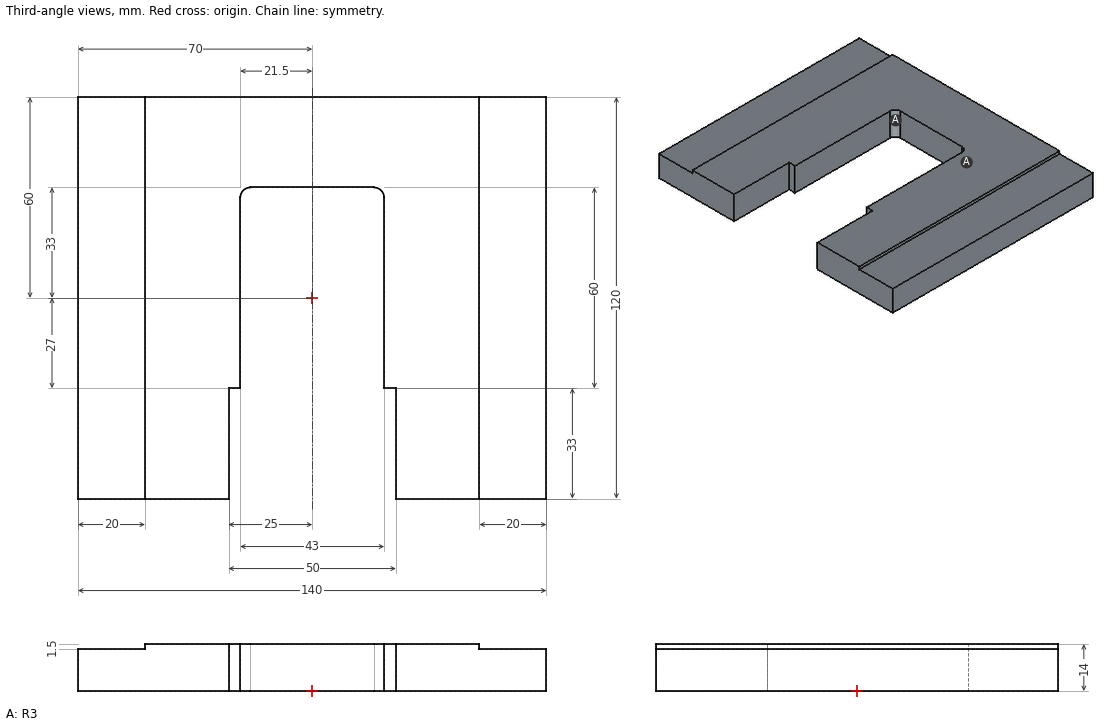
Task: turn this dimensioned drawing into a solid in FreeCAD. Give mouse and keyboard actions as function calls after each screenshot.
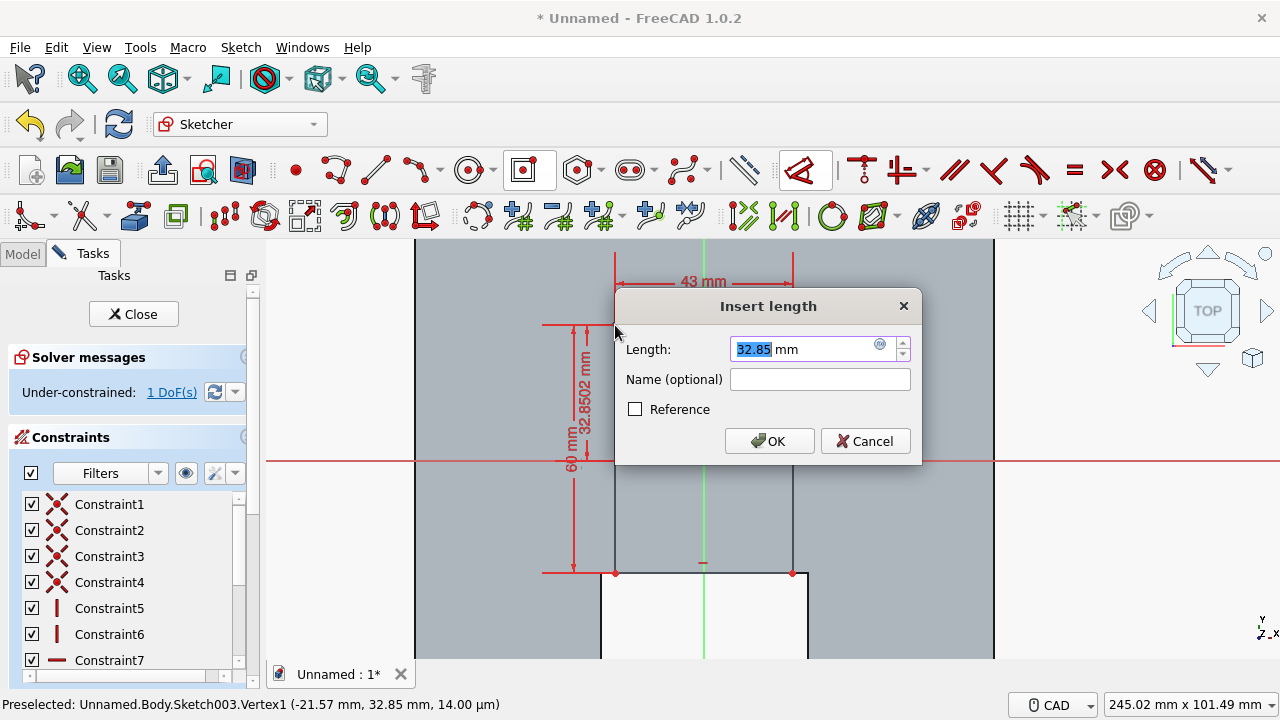
text(33)
key(Return)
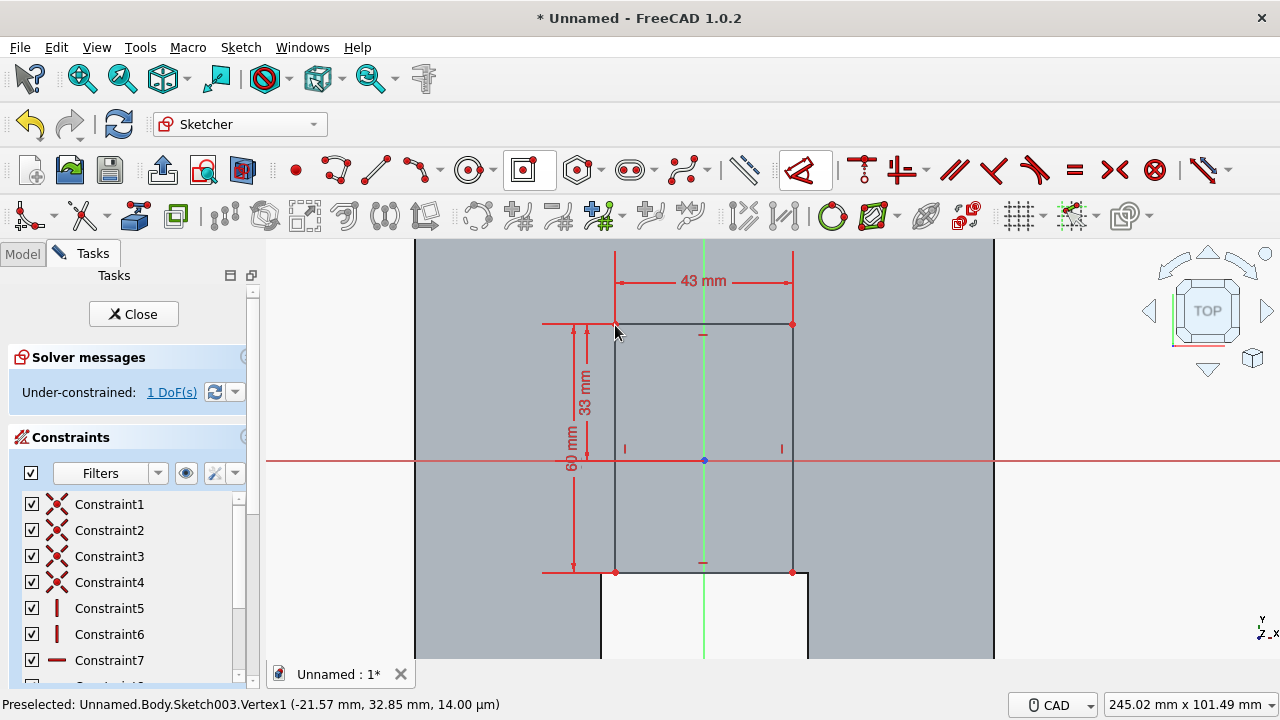
click(615, 324)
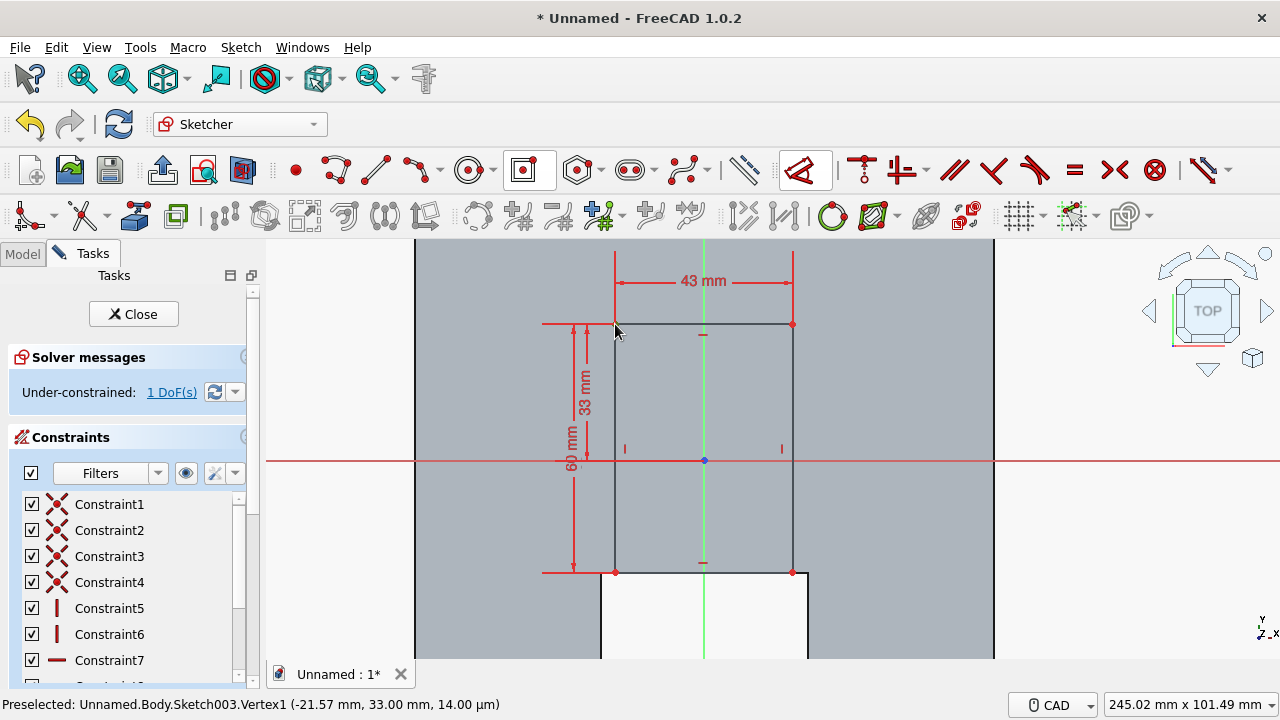
key(l)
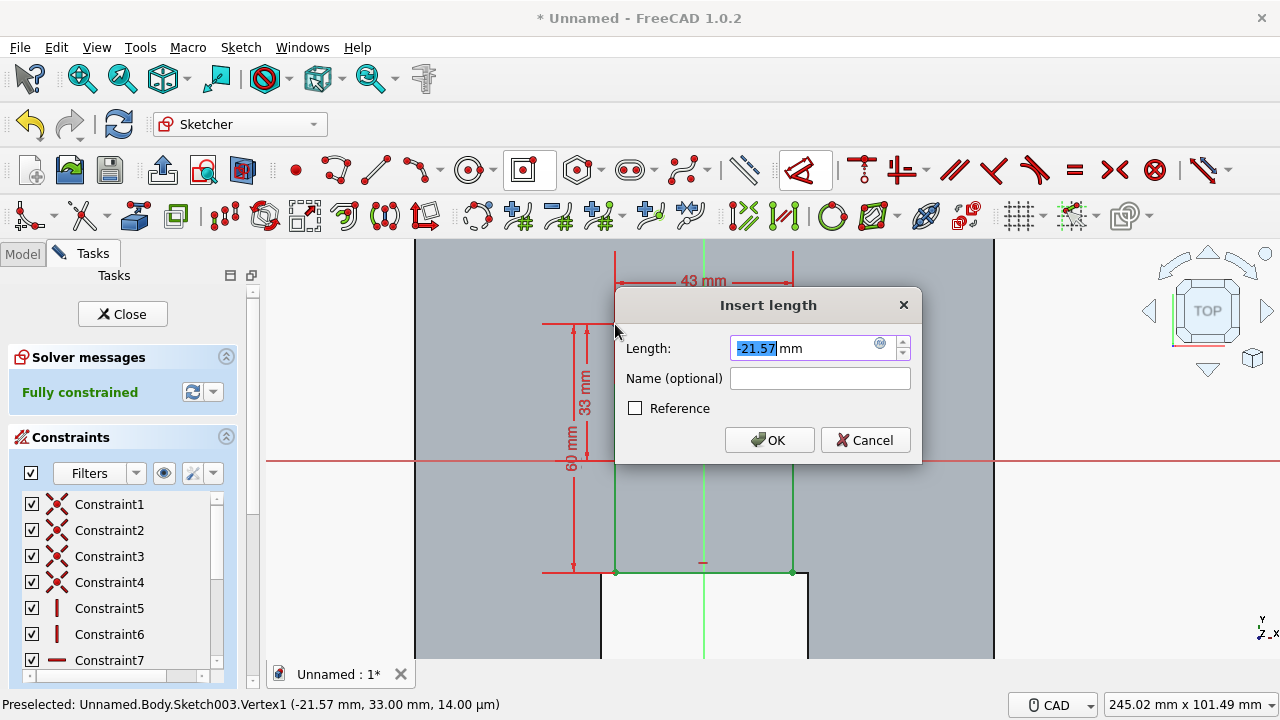
text(-21.5)
key(Return)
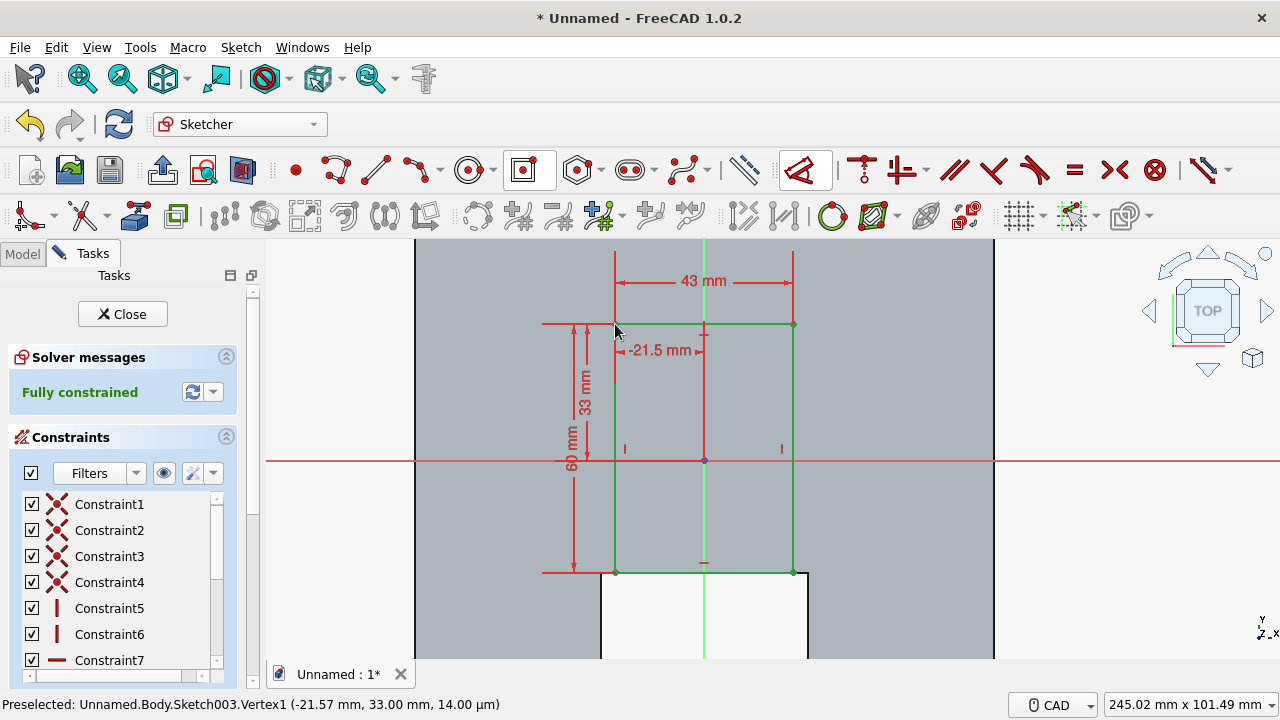
click(123, 314)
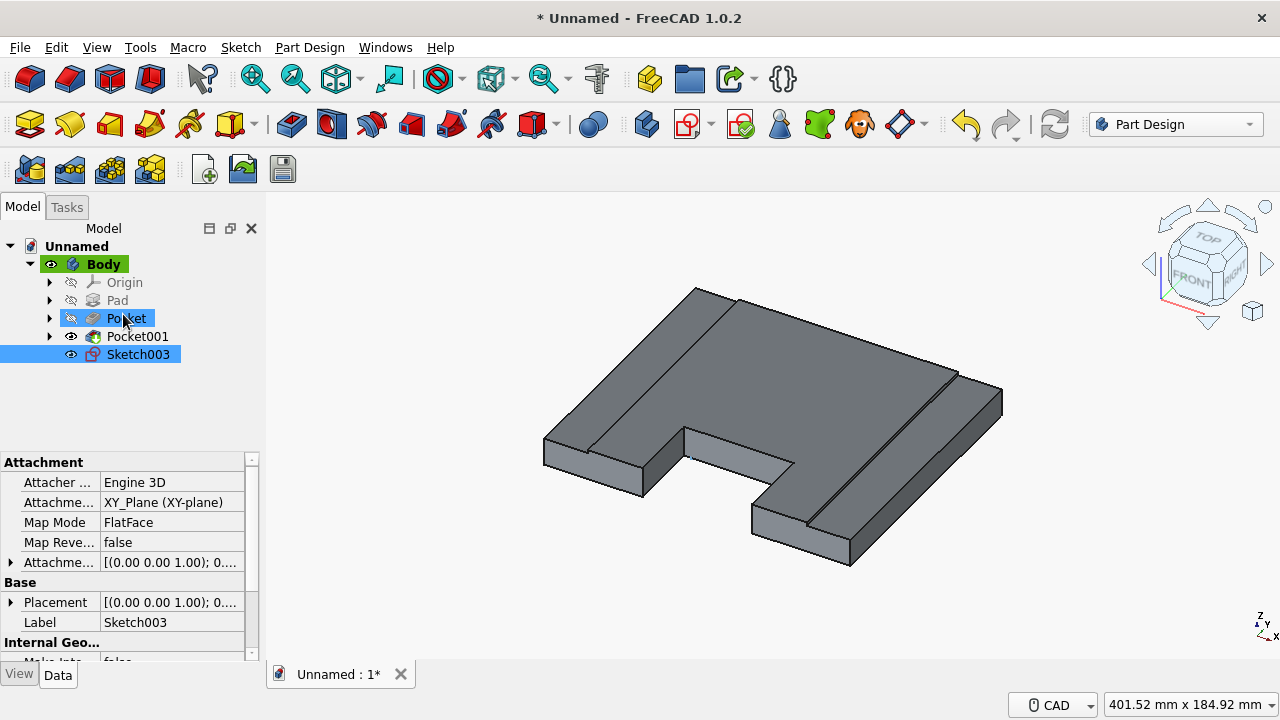
click(292, 124)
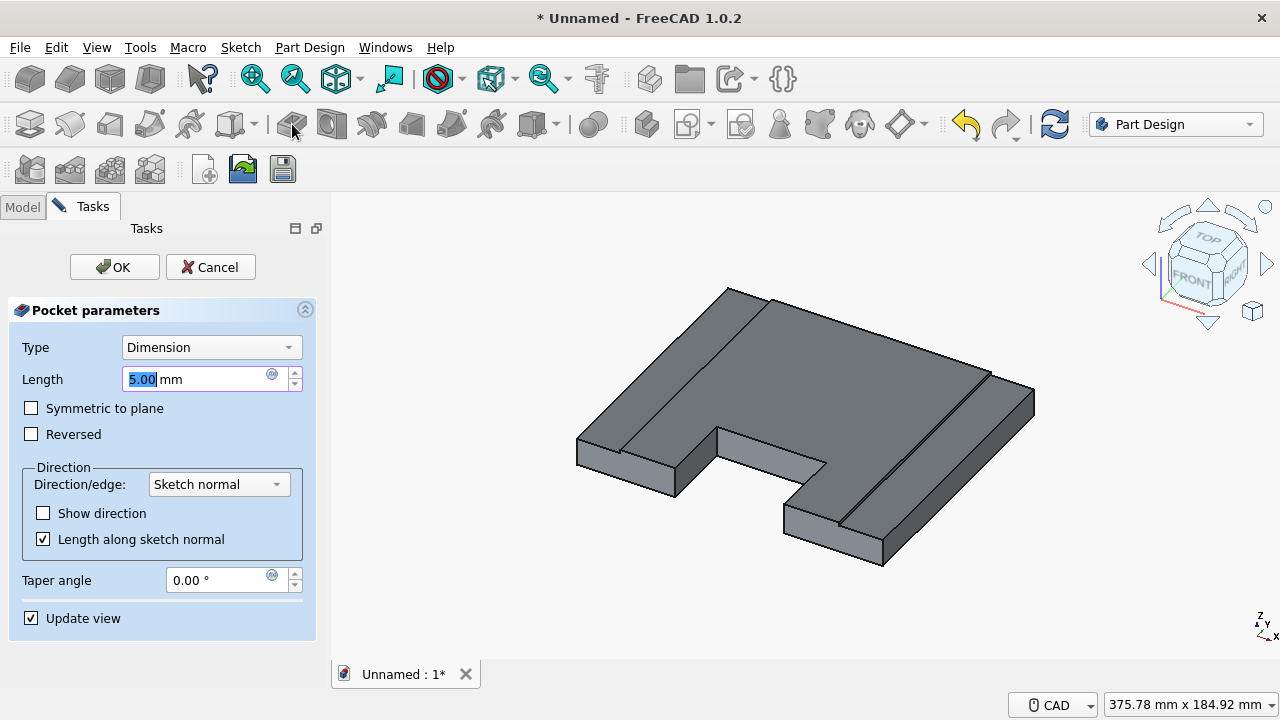
click(212, 348)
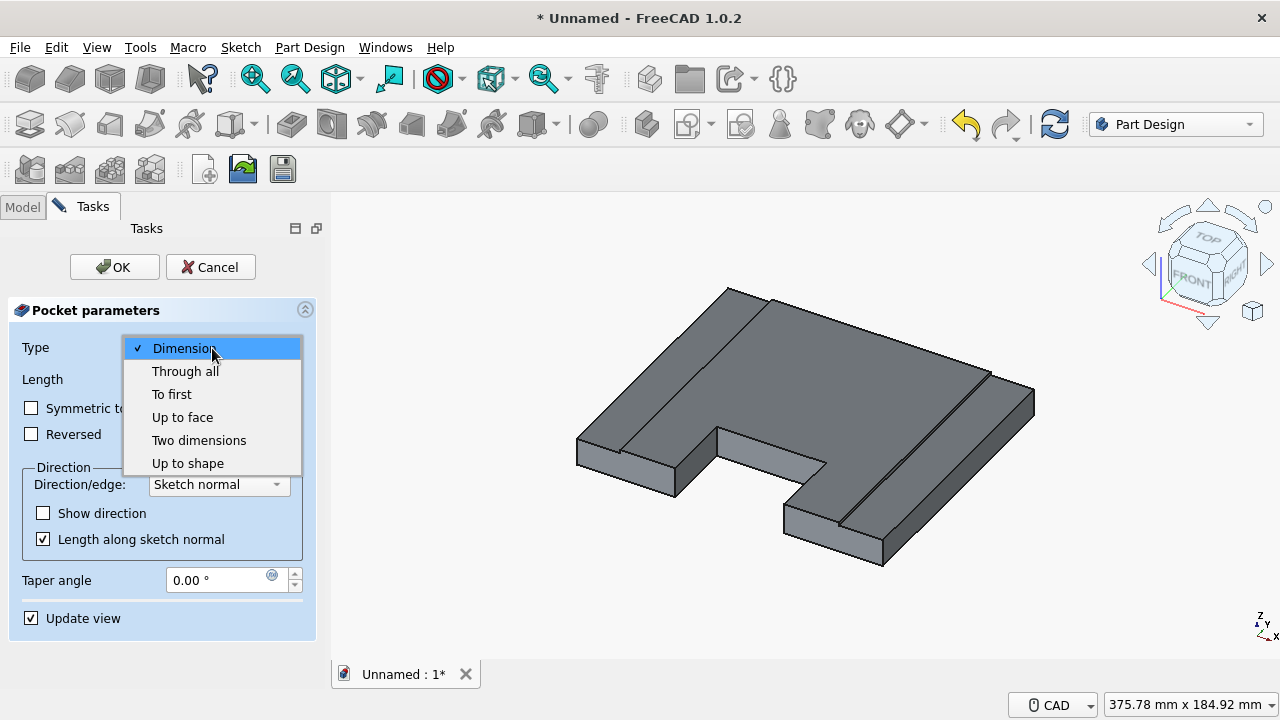
click(212, 394)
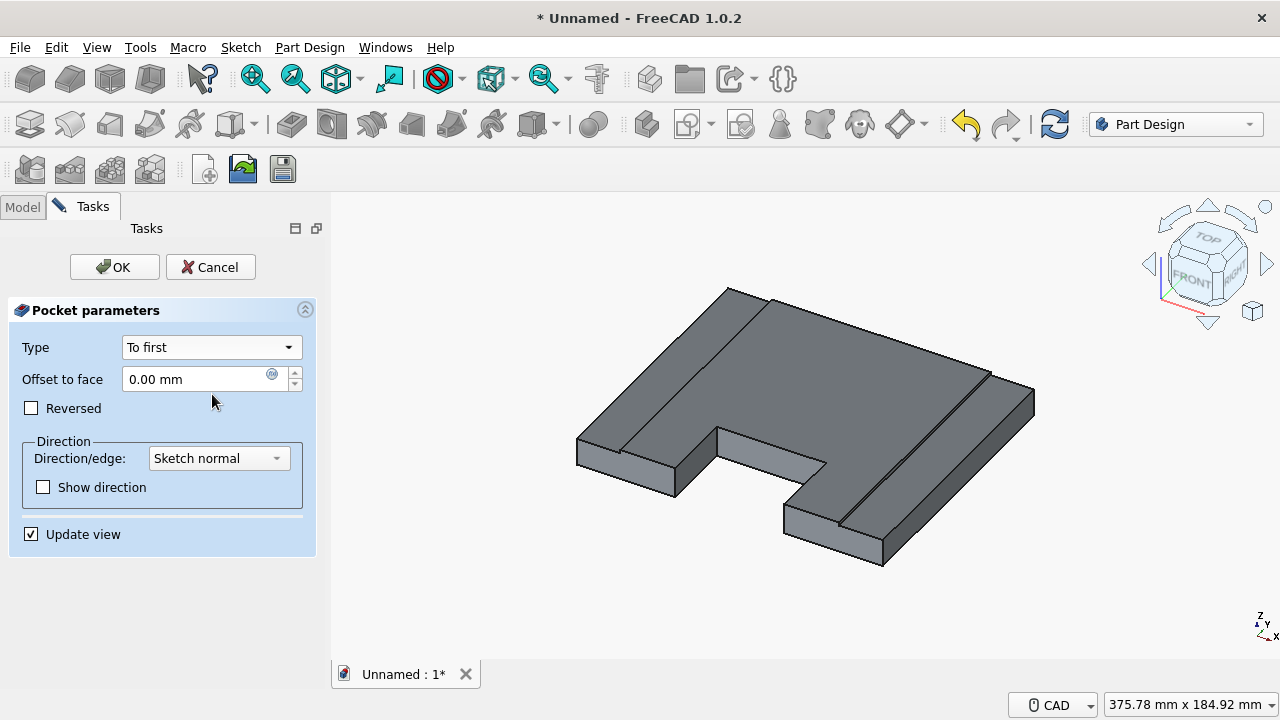
click(30, 408)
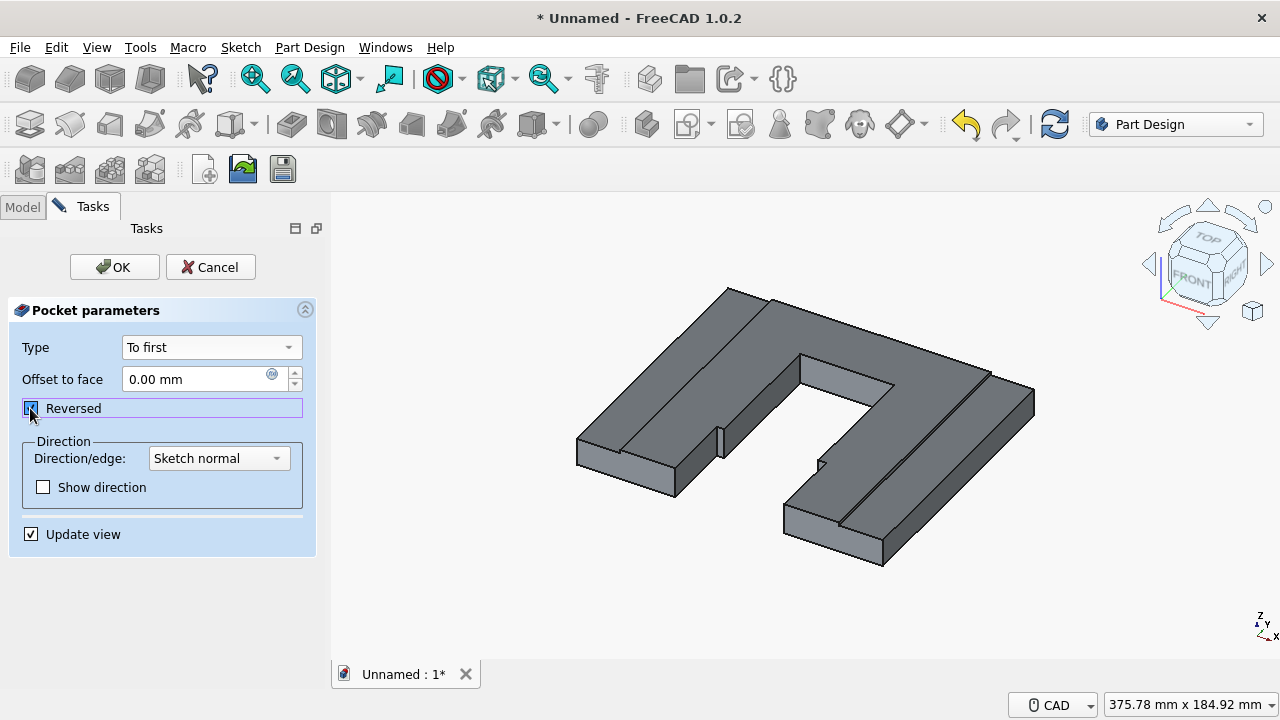
click(115, 267)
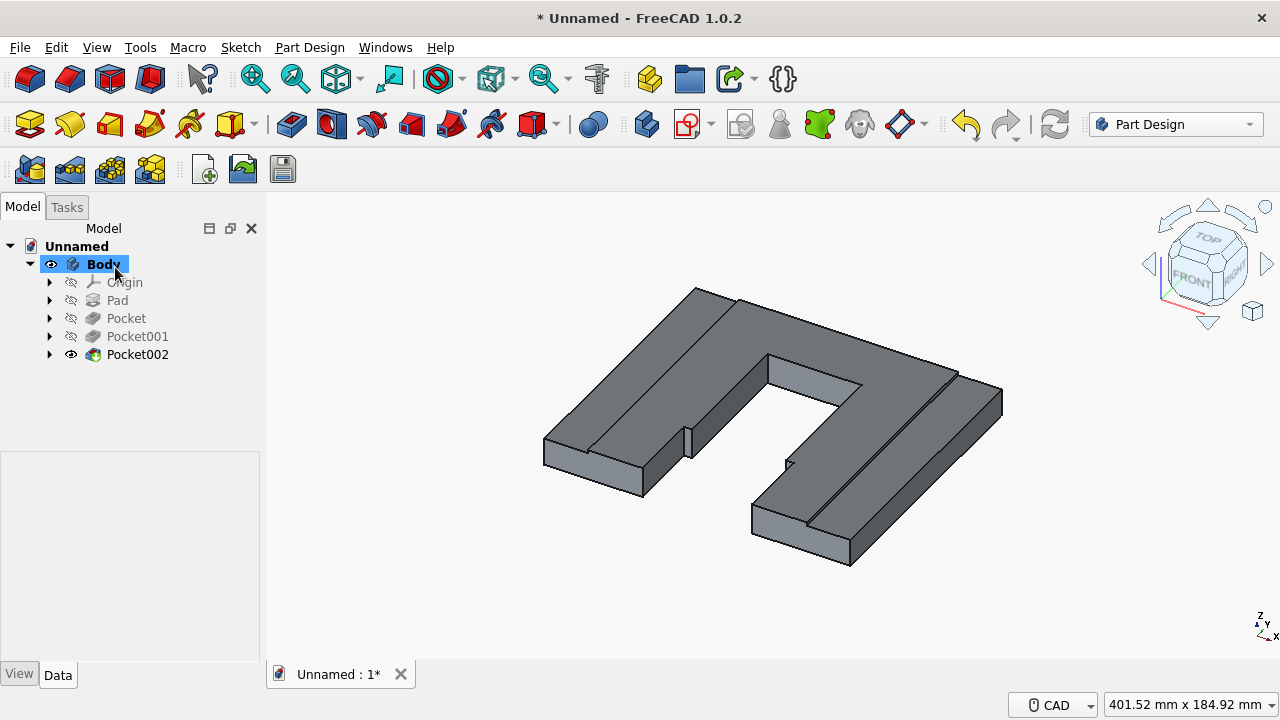
key(0)